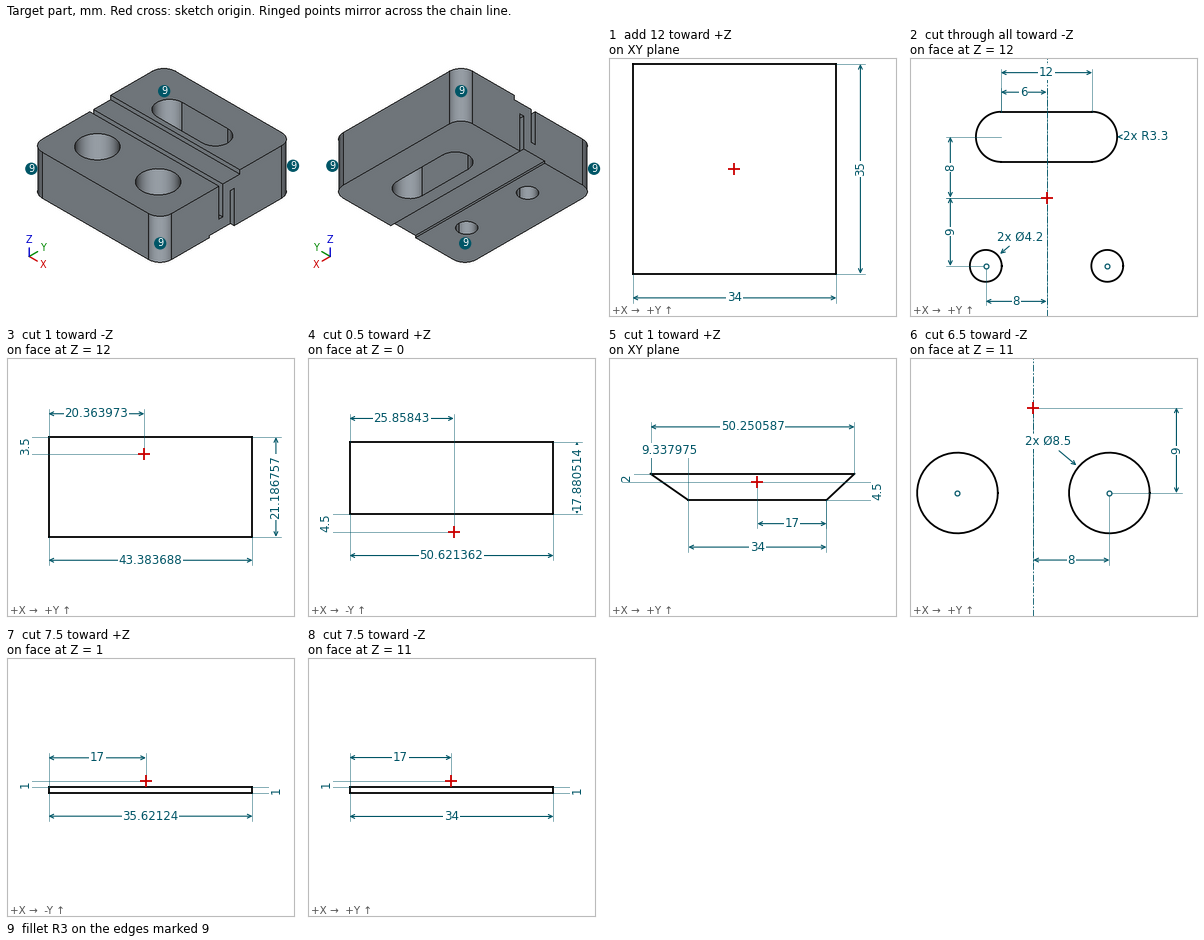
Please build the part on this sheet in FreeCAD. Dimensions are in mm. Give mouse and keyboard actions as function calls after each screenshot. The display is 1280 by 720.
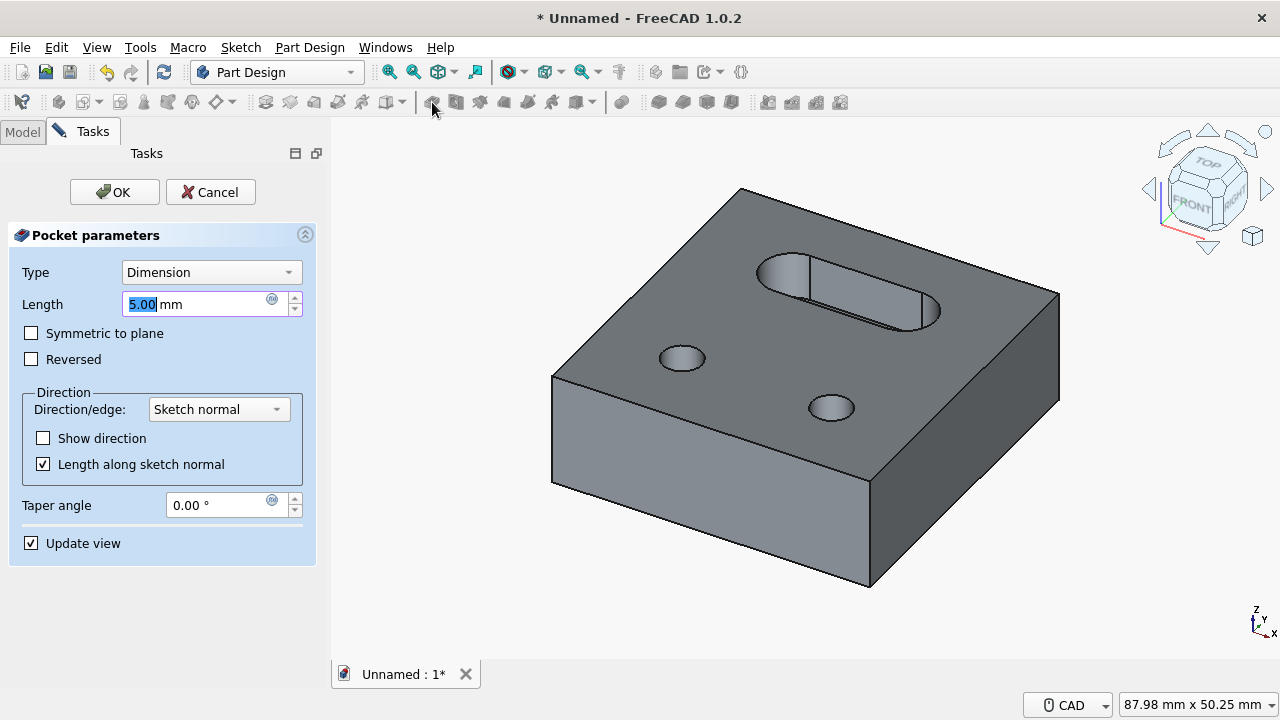
click(212, 272)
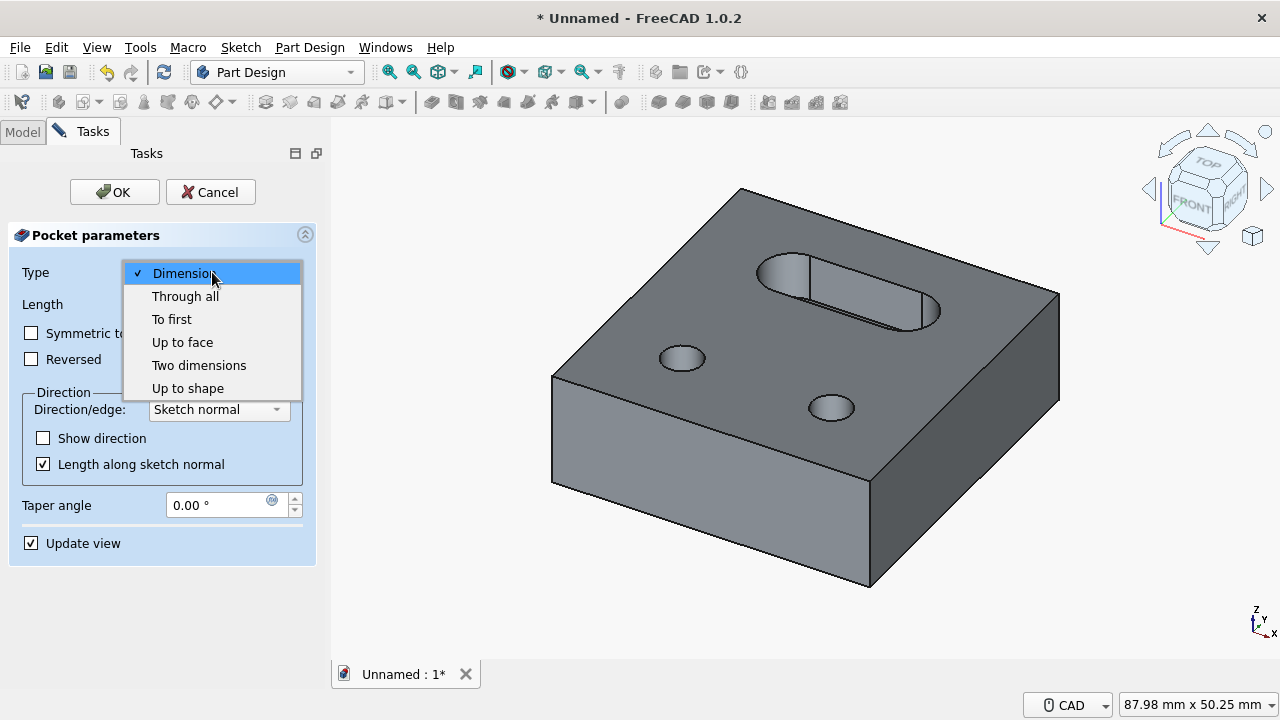
click(212, 296)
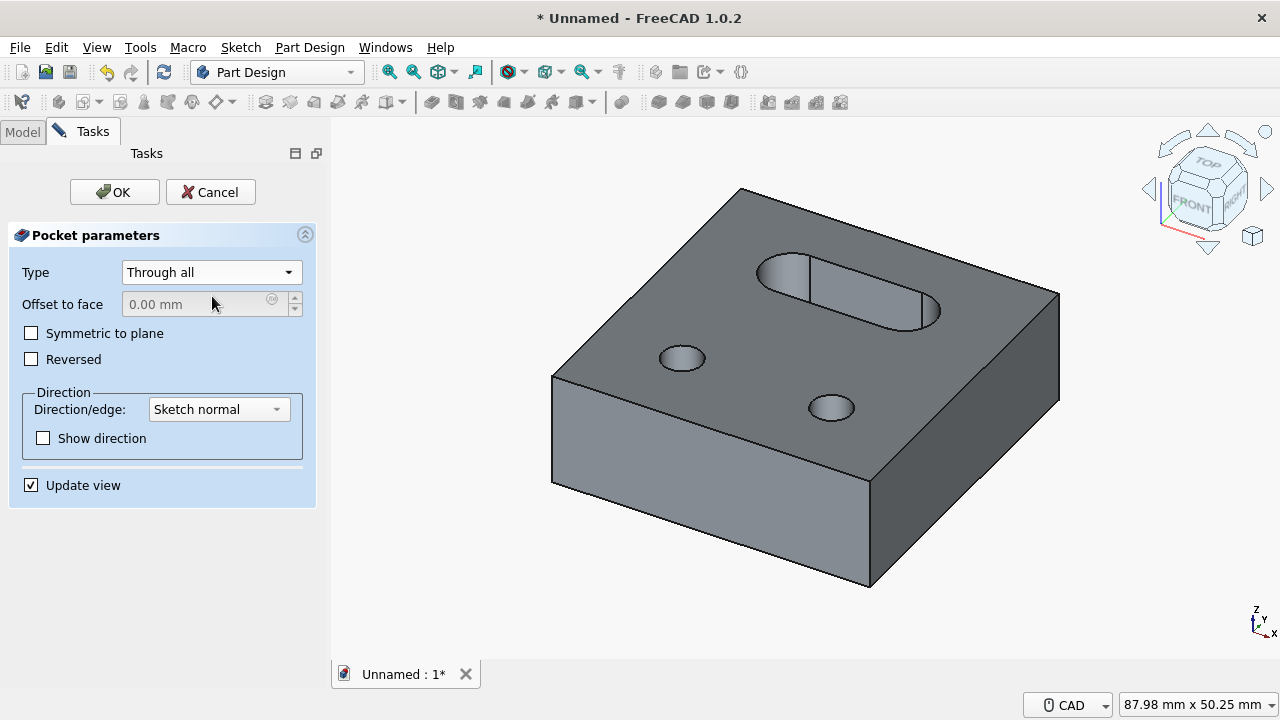
click(115, 192)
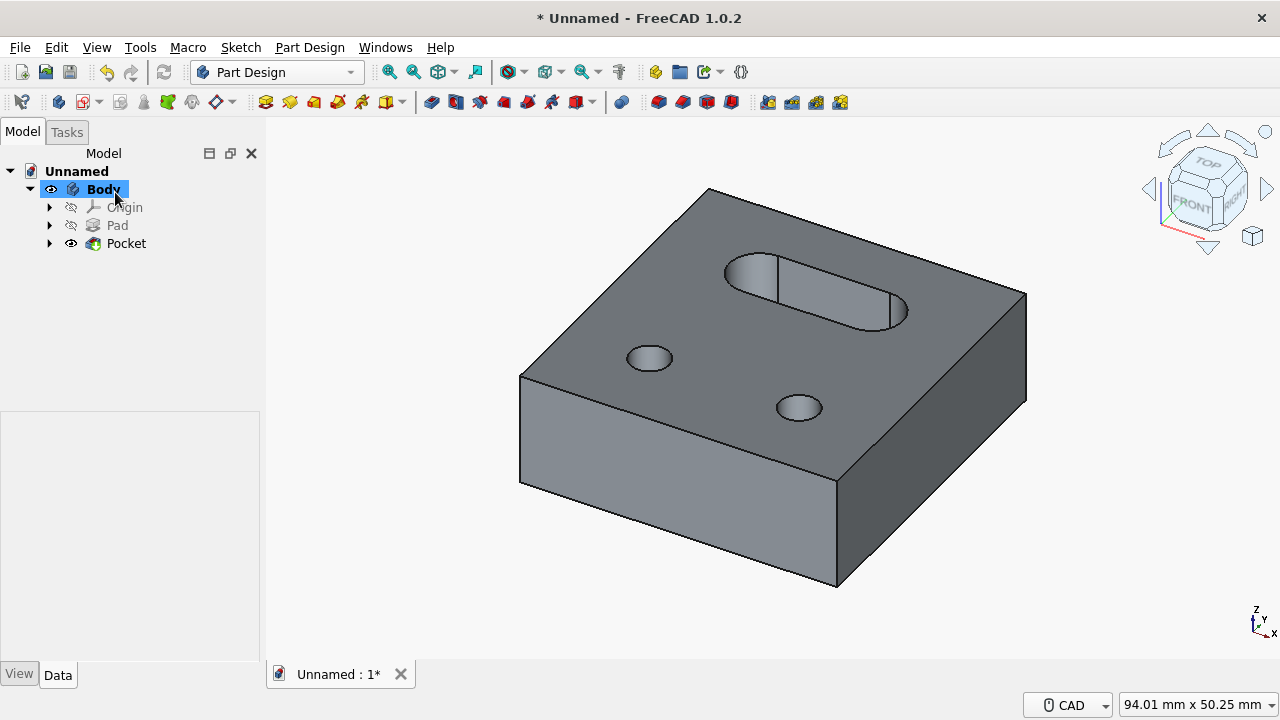
click(746, 361)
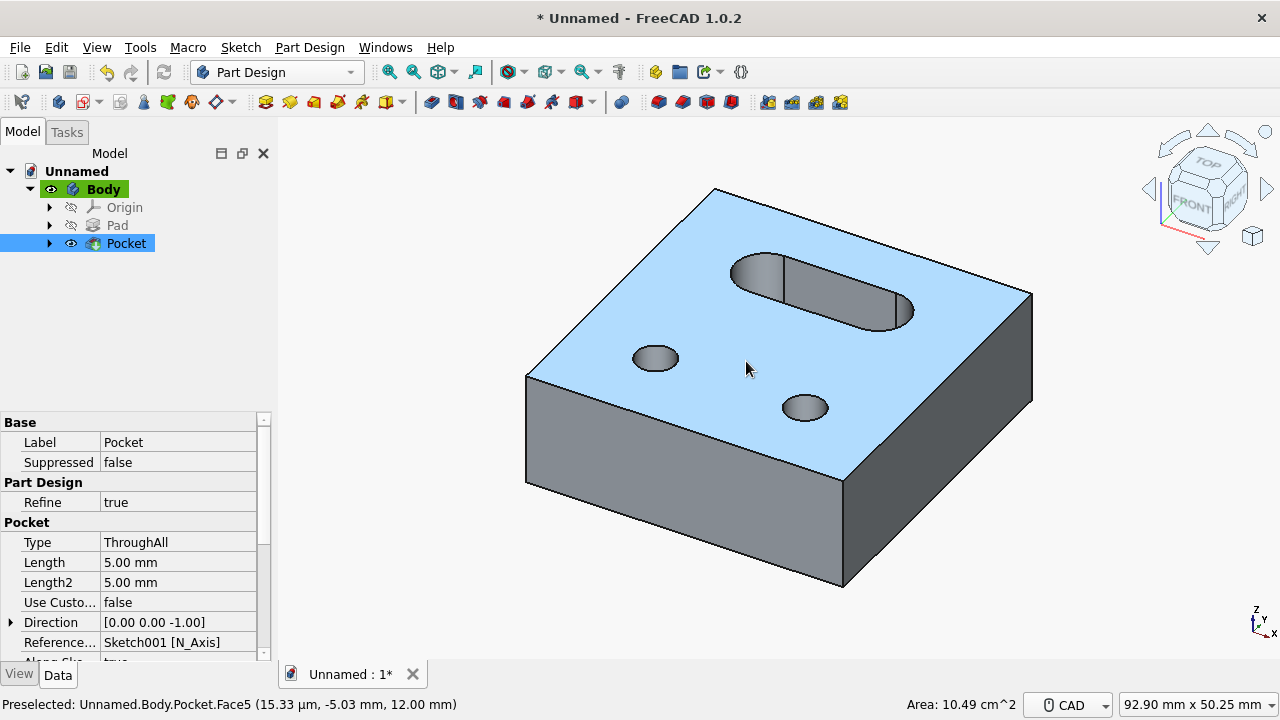
click(84, 102)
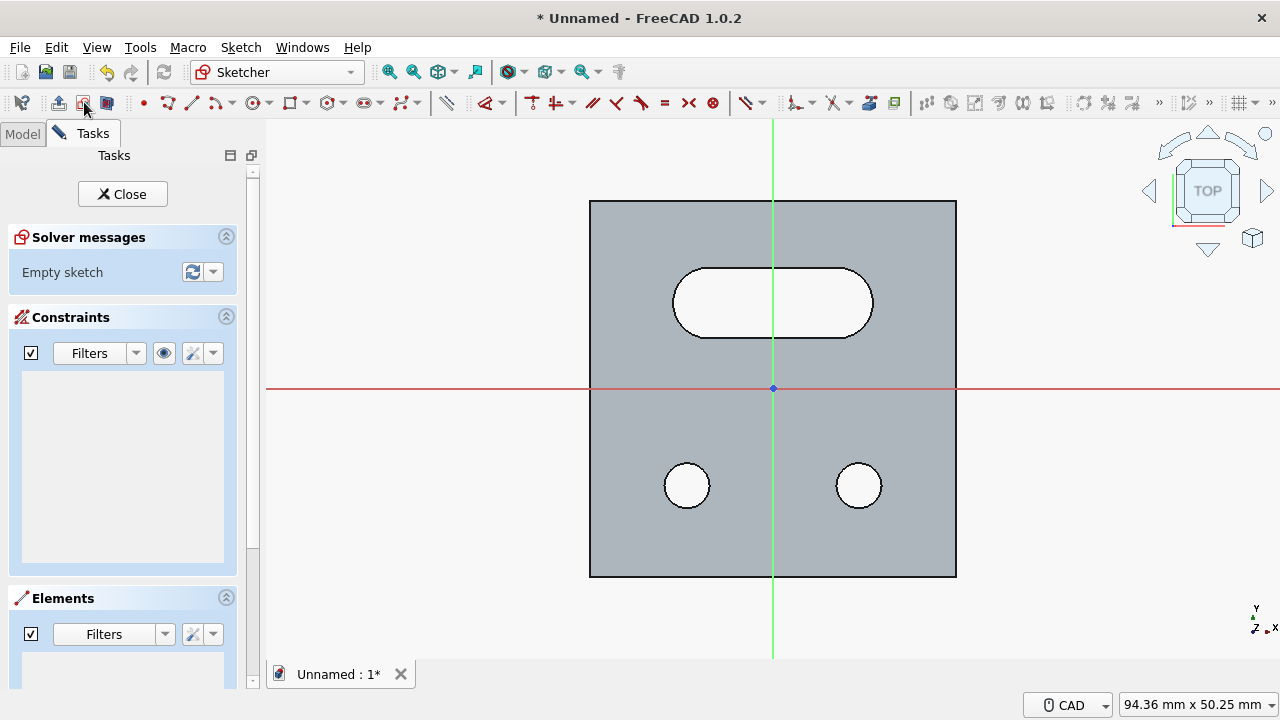
key(g)
key(r)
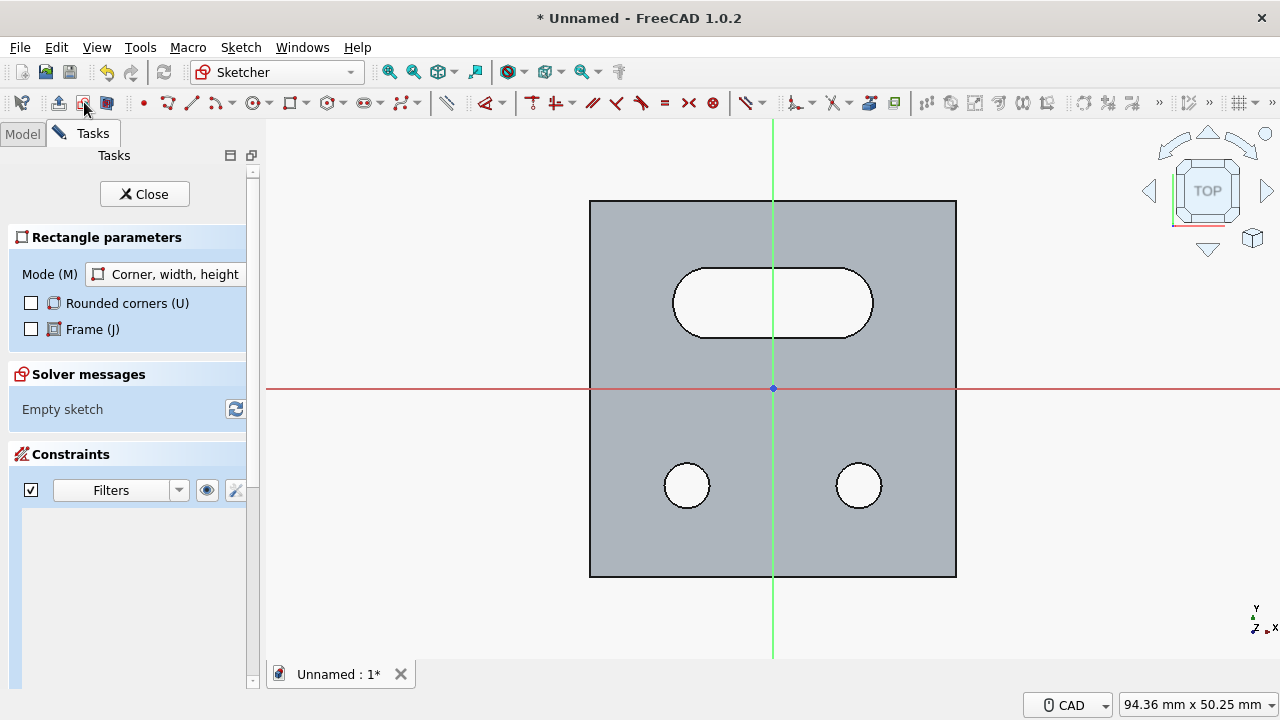
click(554, 351)
move(1020, 579)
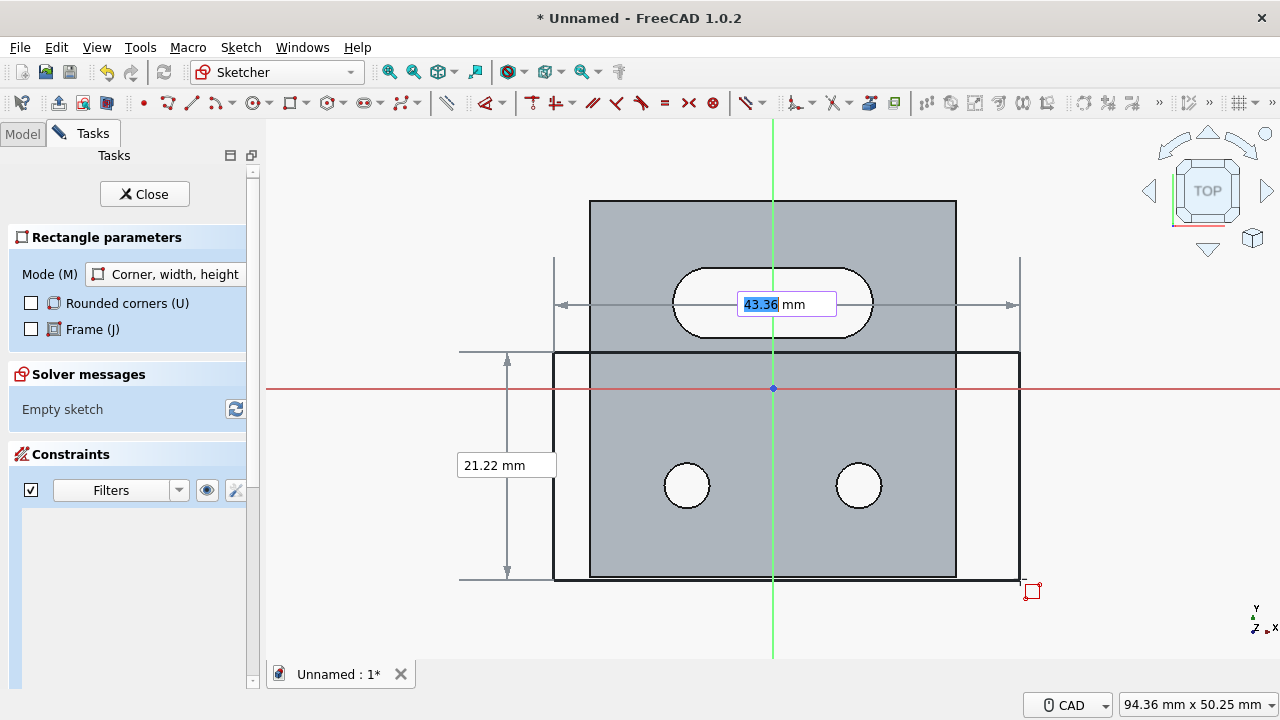
text(43.383688)
key(Tab)
text(21.186757)
key(Return)
key(Escape)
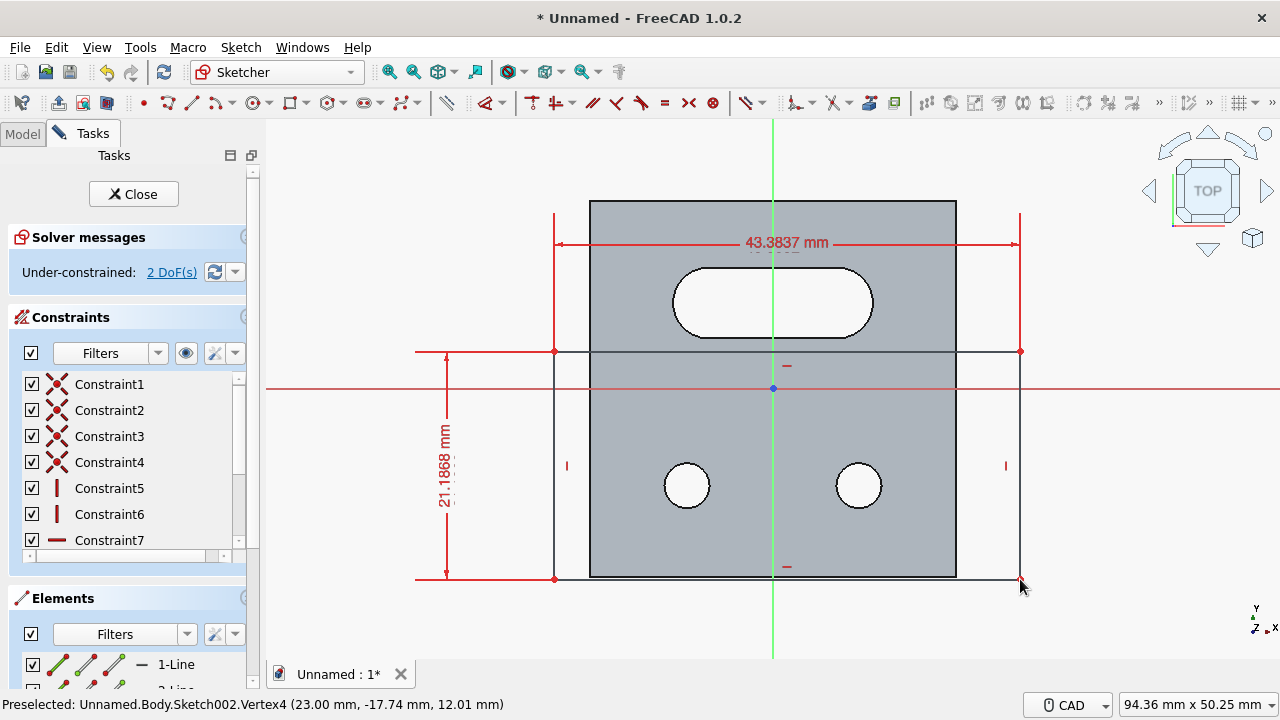
key(d)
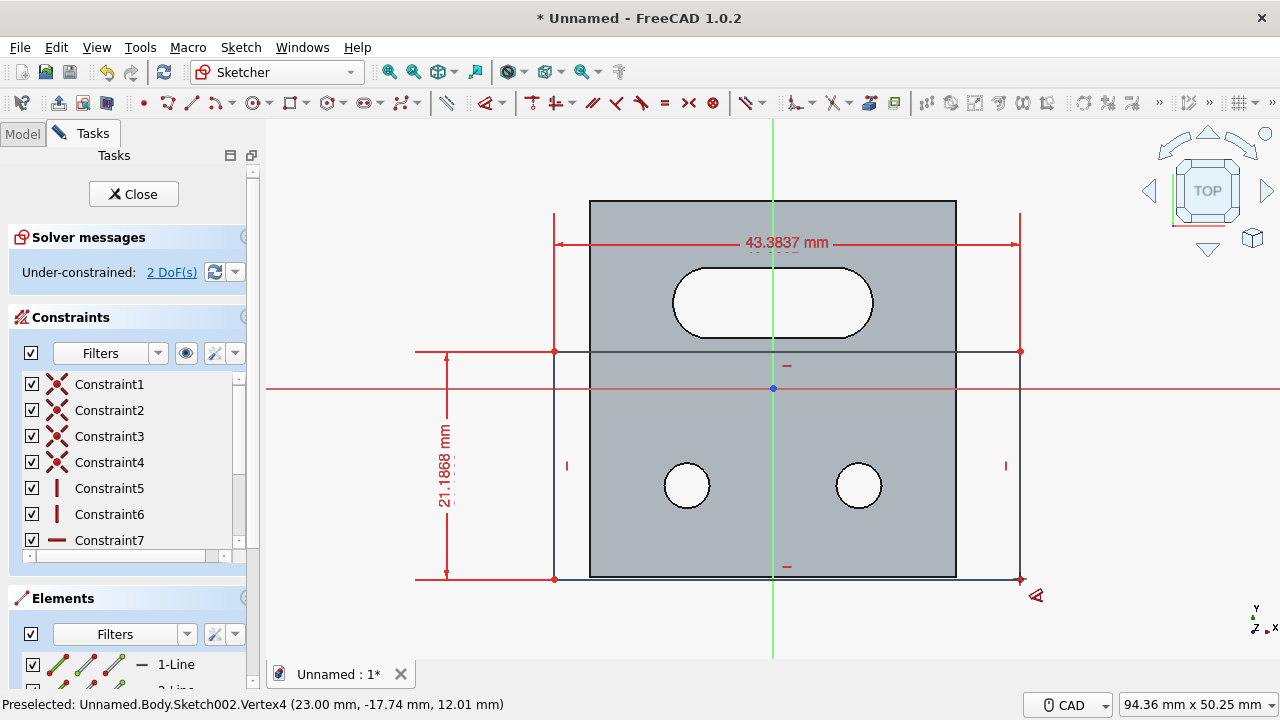
click(554, 352)
click(520, 370)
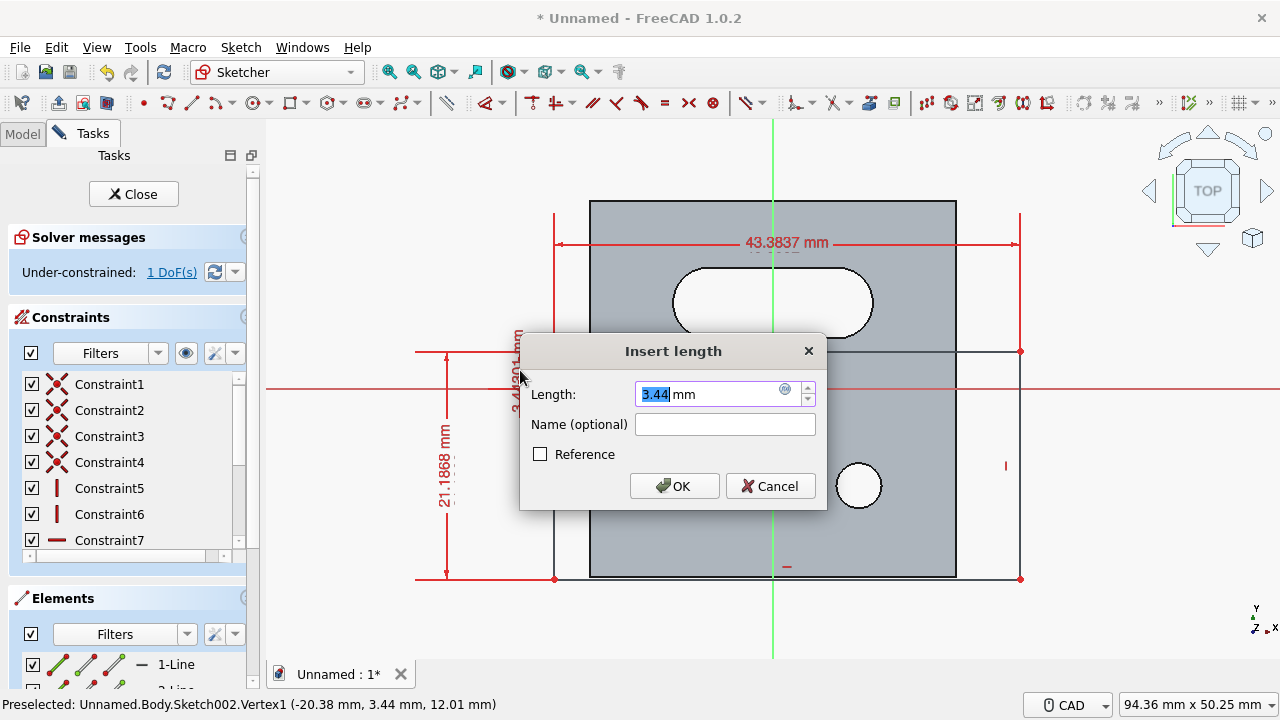
text(3.5)
key(Return)